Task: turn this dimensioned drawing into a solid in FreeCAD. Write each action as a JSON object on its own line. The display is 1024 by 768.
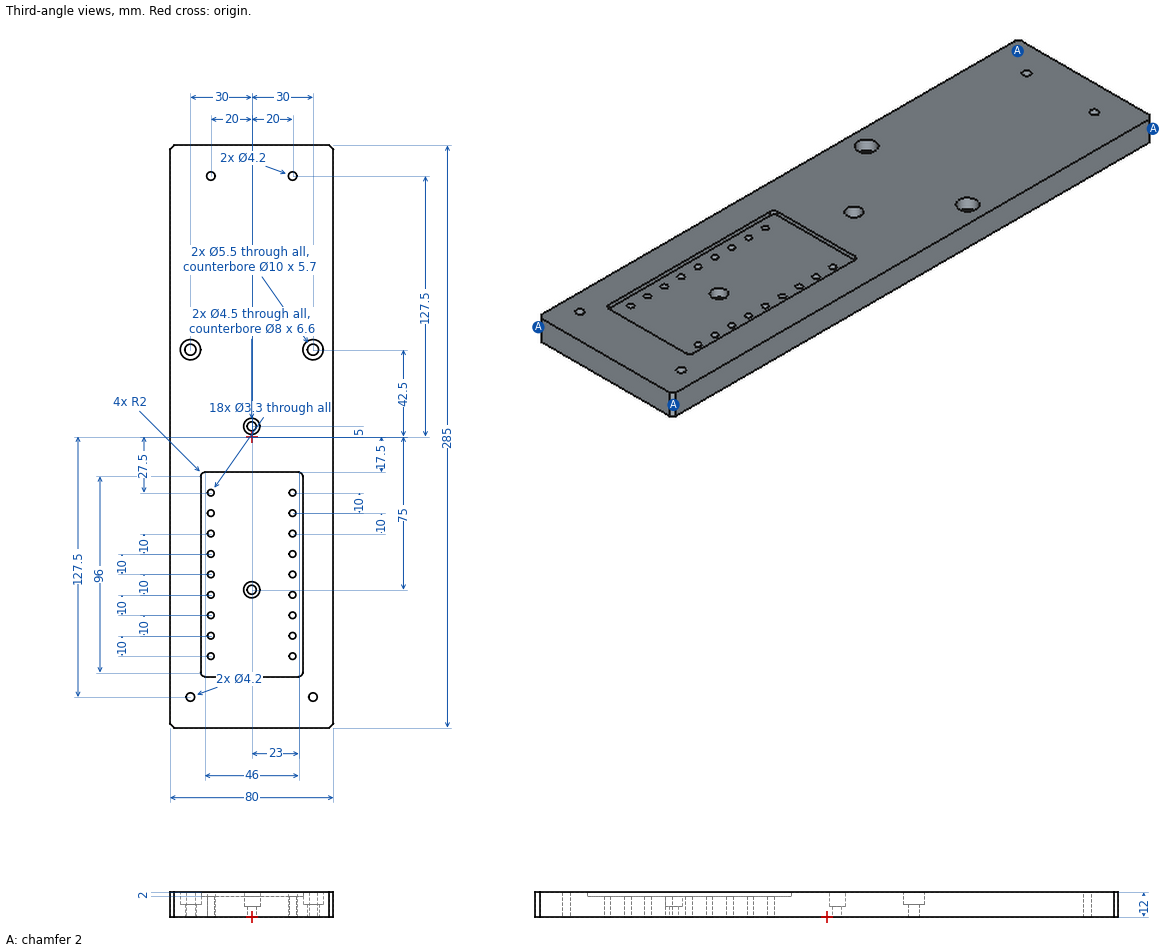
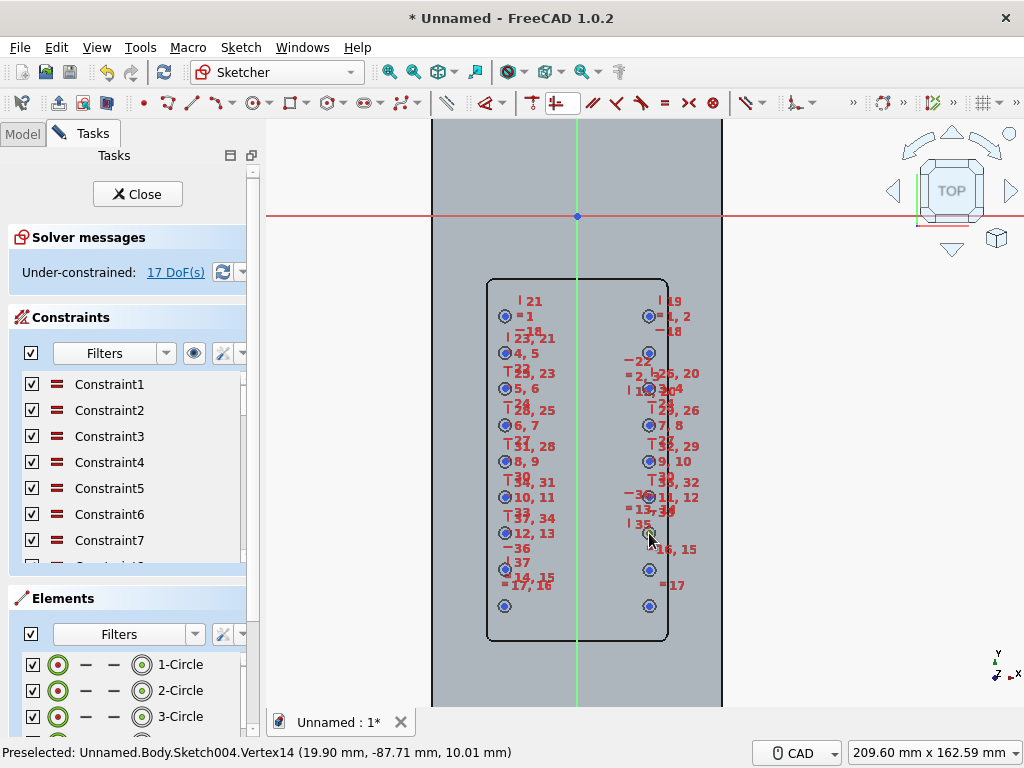
{"action": "left_click", "coordinate": [650, 570]}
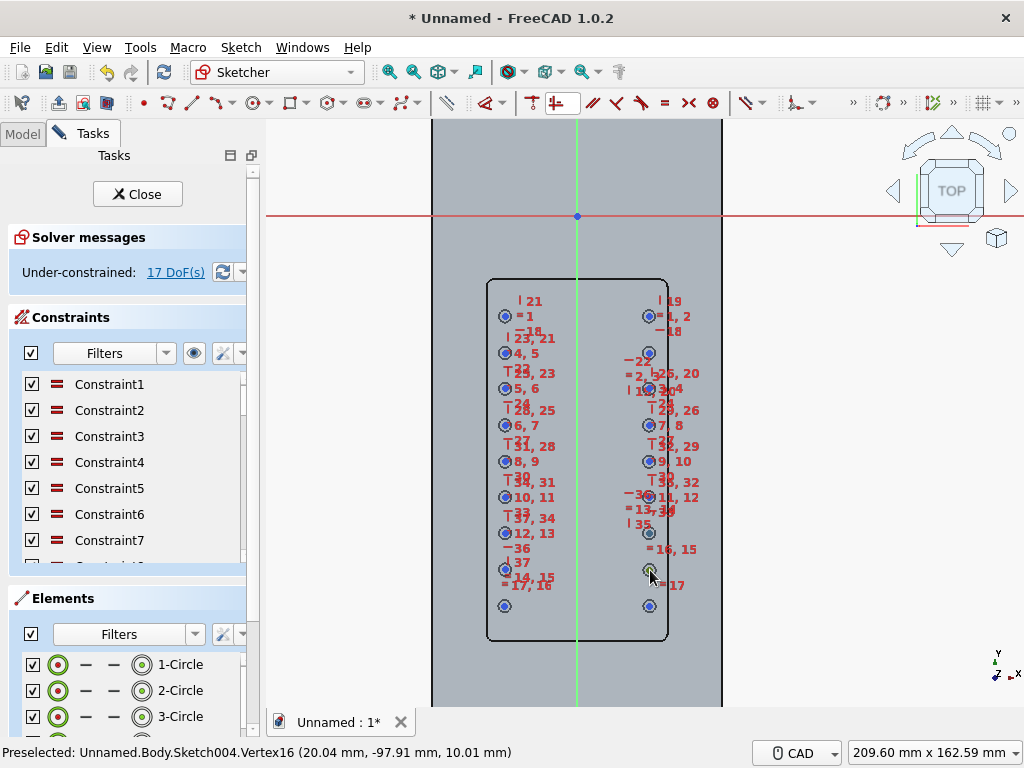
{"action": "key", "text": "v"}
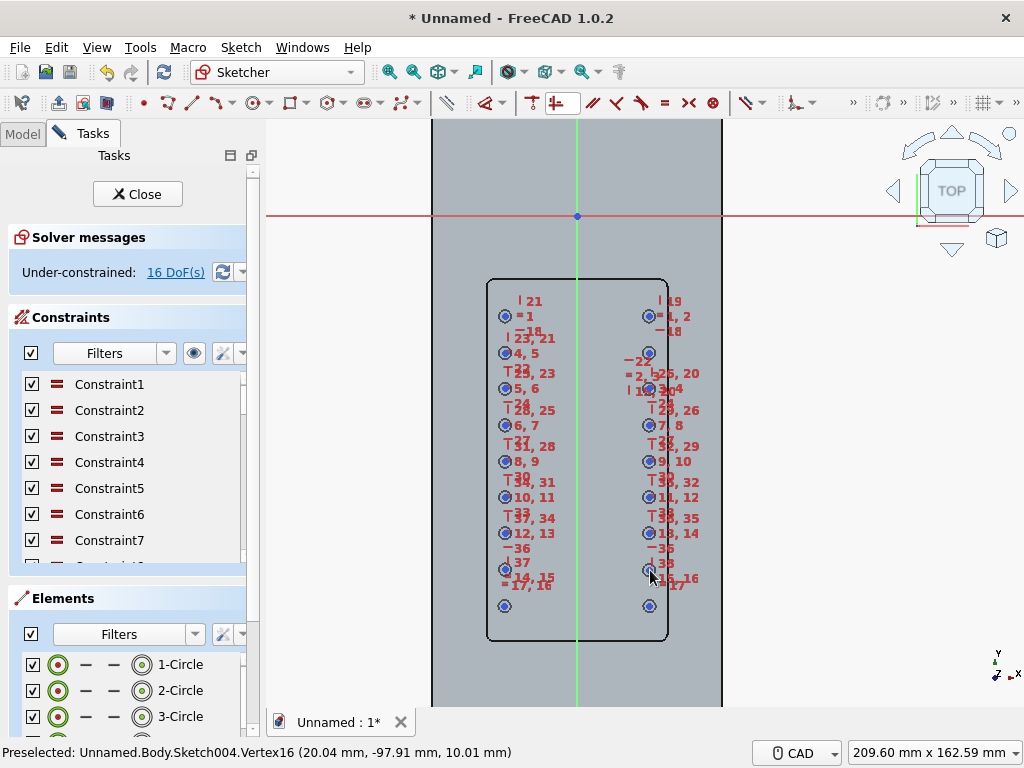
{"action": "scroll", "coordinate": [505, 570], "scroll_direction": "up", "scroll_amount": 4}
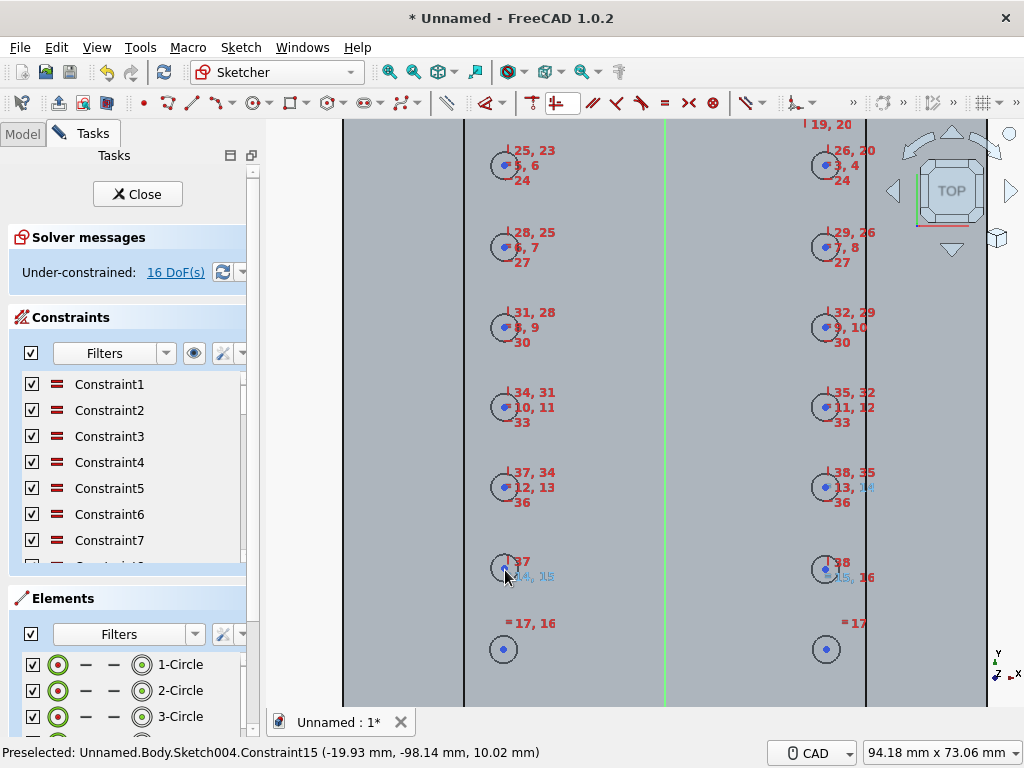
{"action": "scroll", "coordinate": [505, 568], "scroll_direction": "up", "scroll_amount": 4}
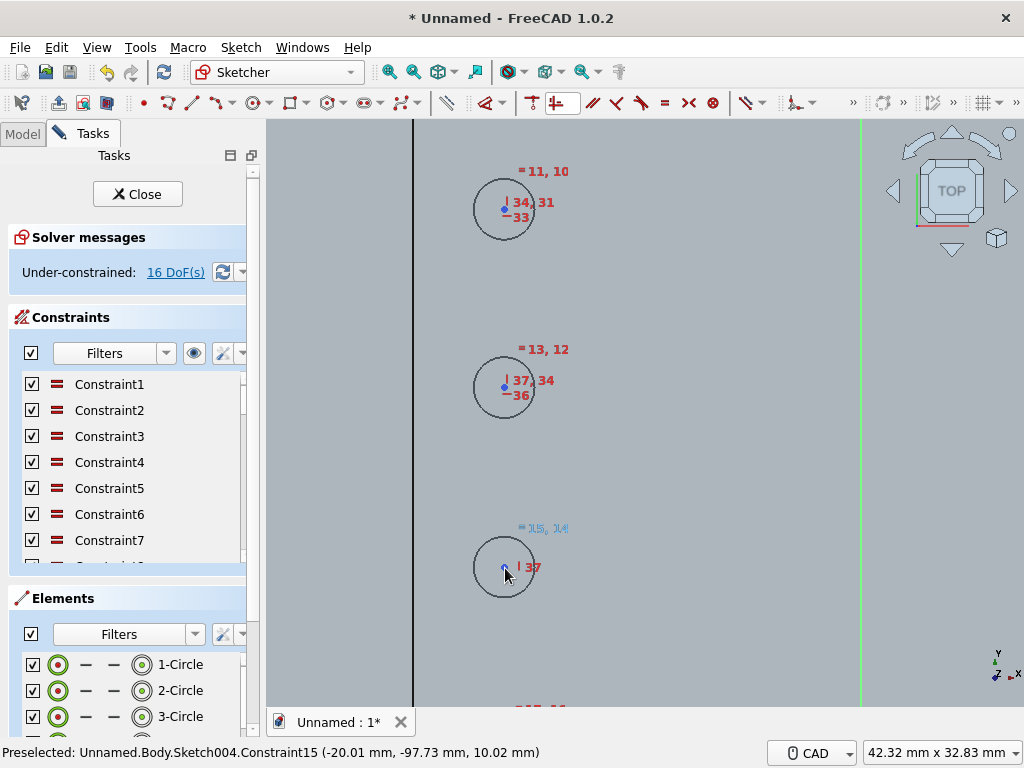
{"action": "left_click", "coordinate": [504, 567]}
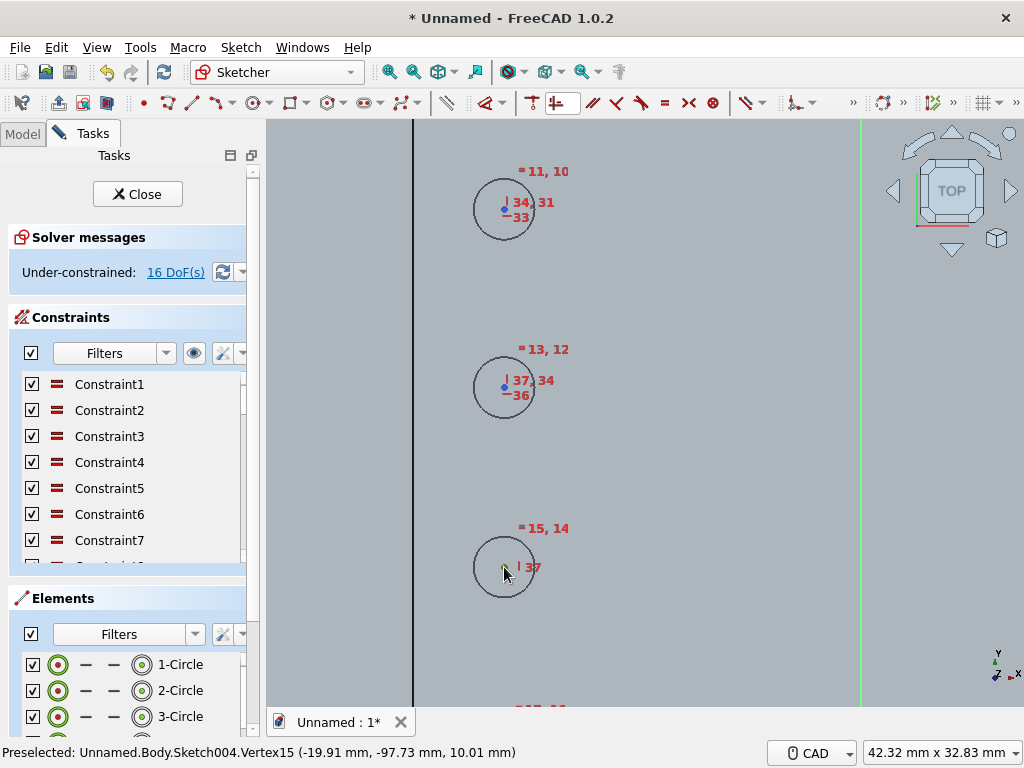
{"action": "scroll", "coordinate": [505, 570], "scroll_direction": "down", "scroll_amount": 8}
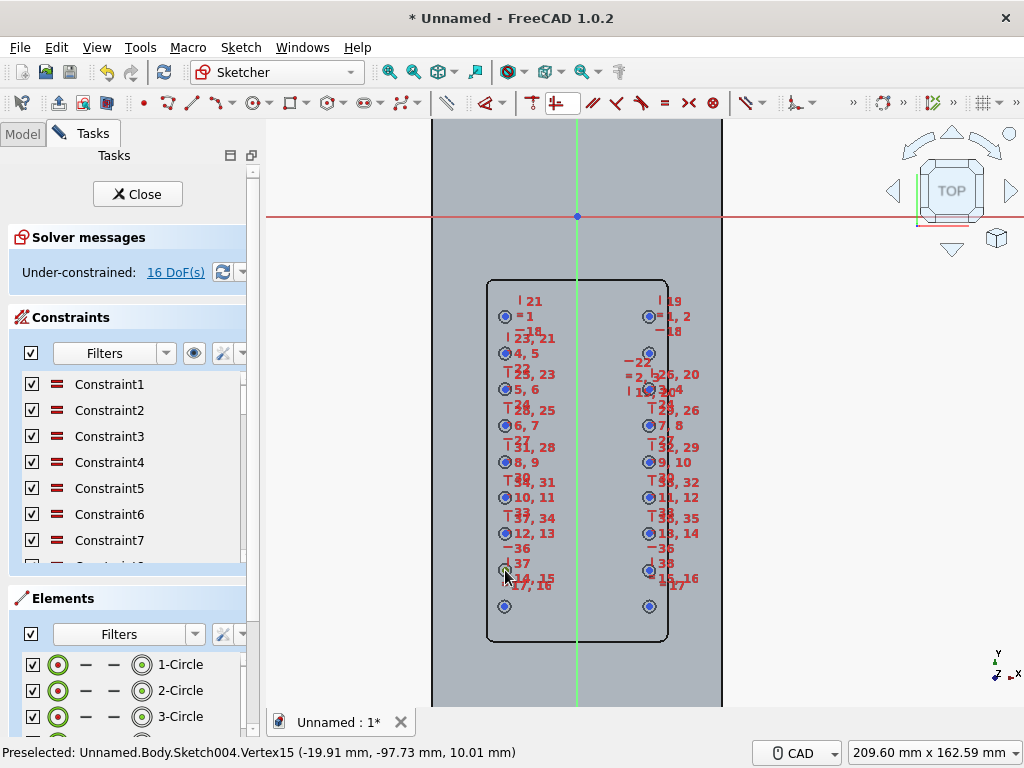
{"action": "scroll", "coordinate": [649, 571], "scroll_direction": "up", "scroll_amount": 4}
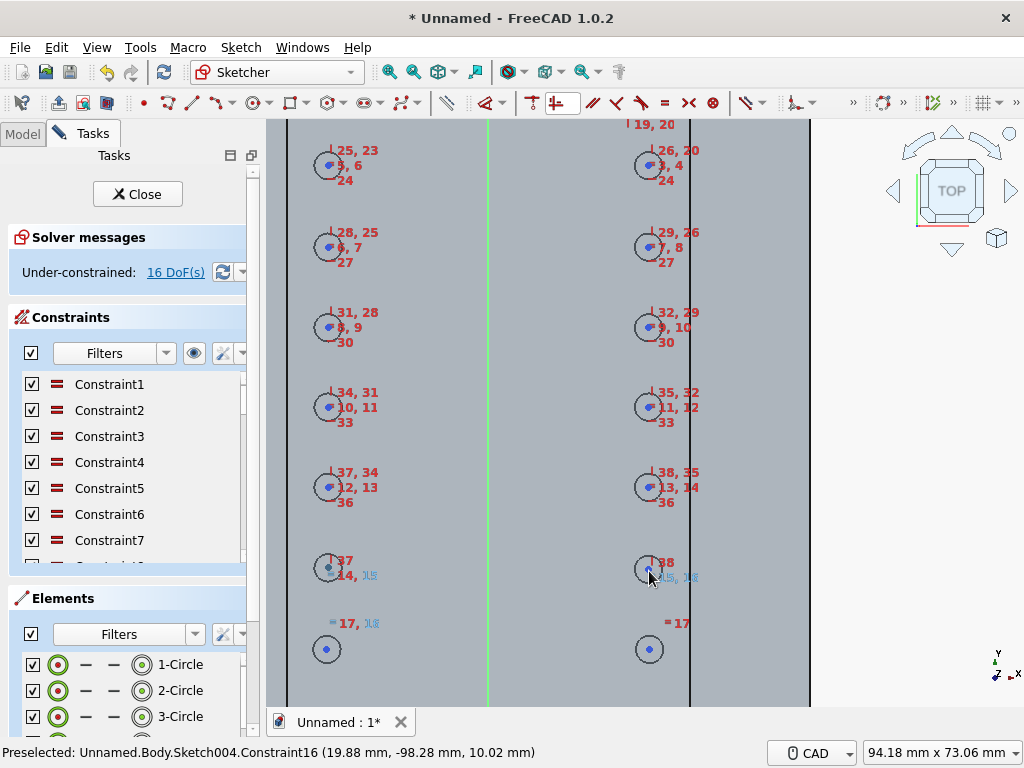
{"action": "scroll", "coordinate": [649, 569], "scroll_direction": "up", "scroll_amount": 4}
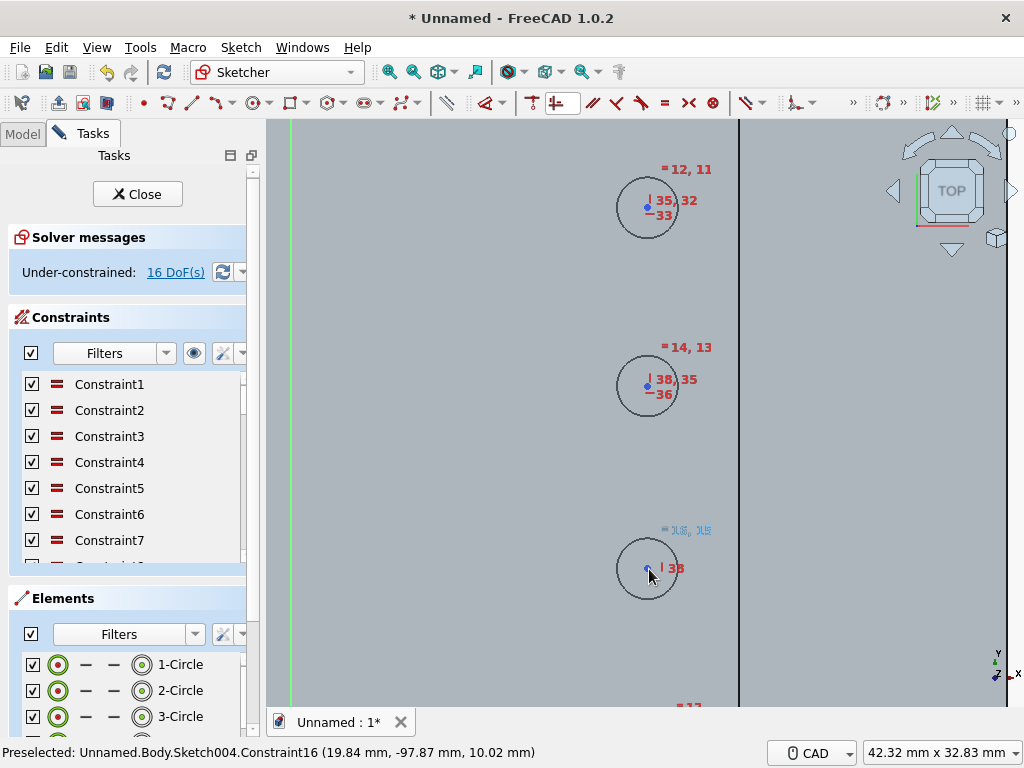
{"action": "left_click", "coordinate": [647, 569]}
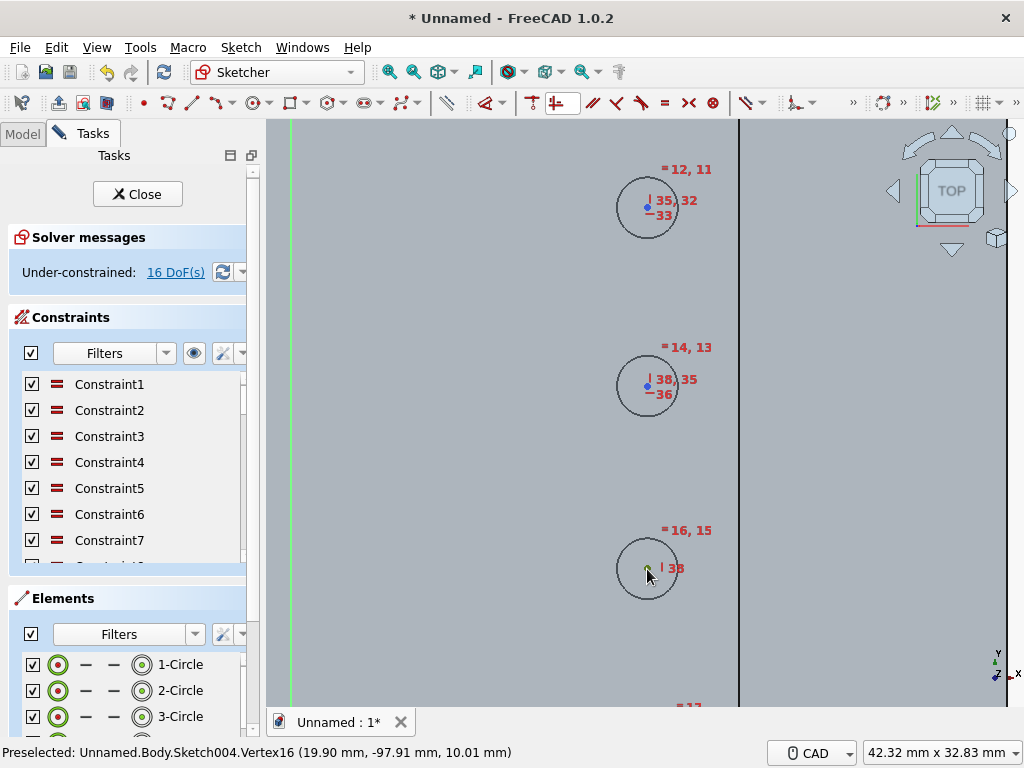
{"action": "left_click", "coordinate": [574, 104]}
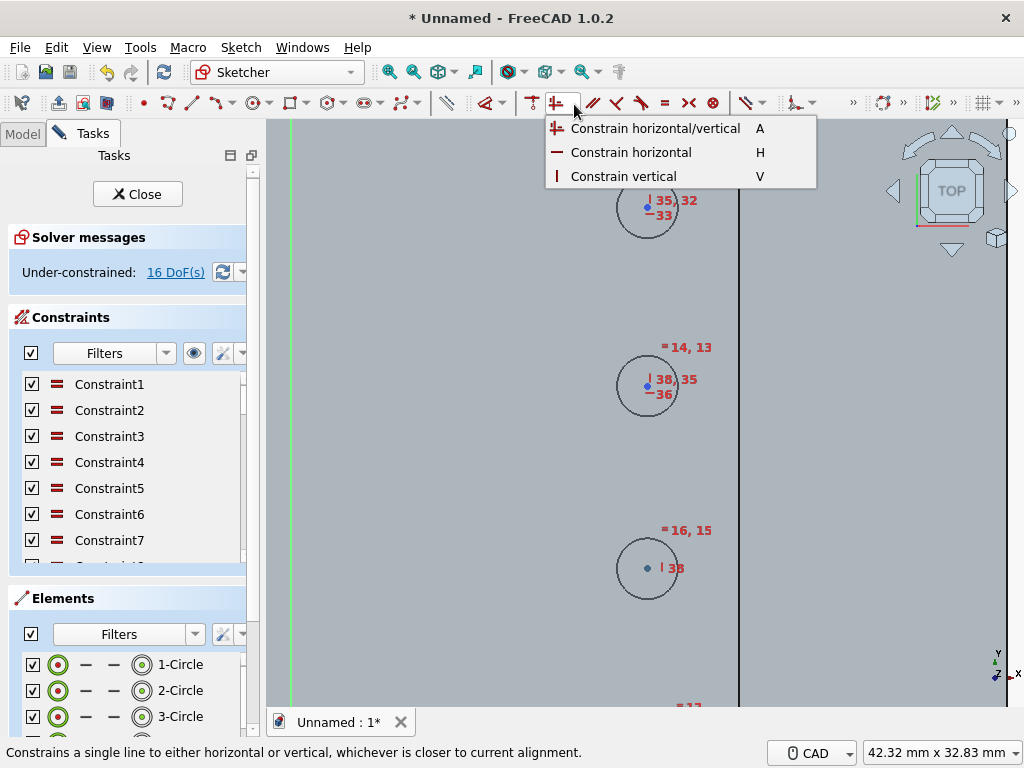
{"action": "left_click", "coordinate": [681, 152]}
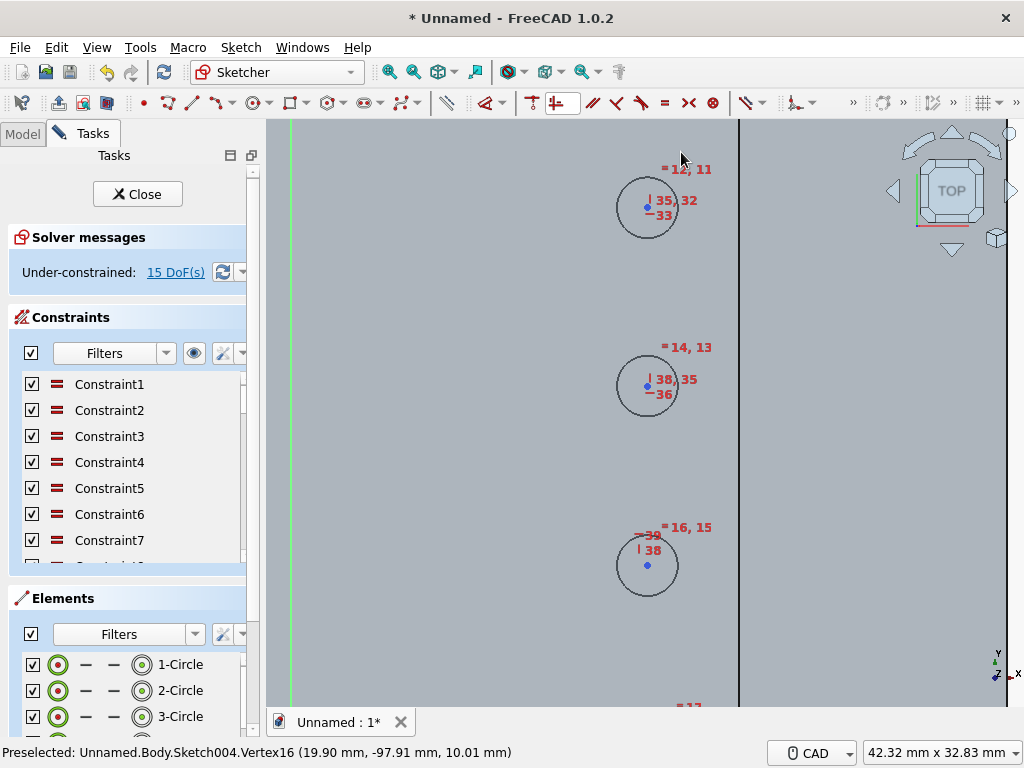
{"action": "scroll", "coordinate": [649, 570], "scroll_direction": "down", "scroll_amount": 8}